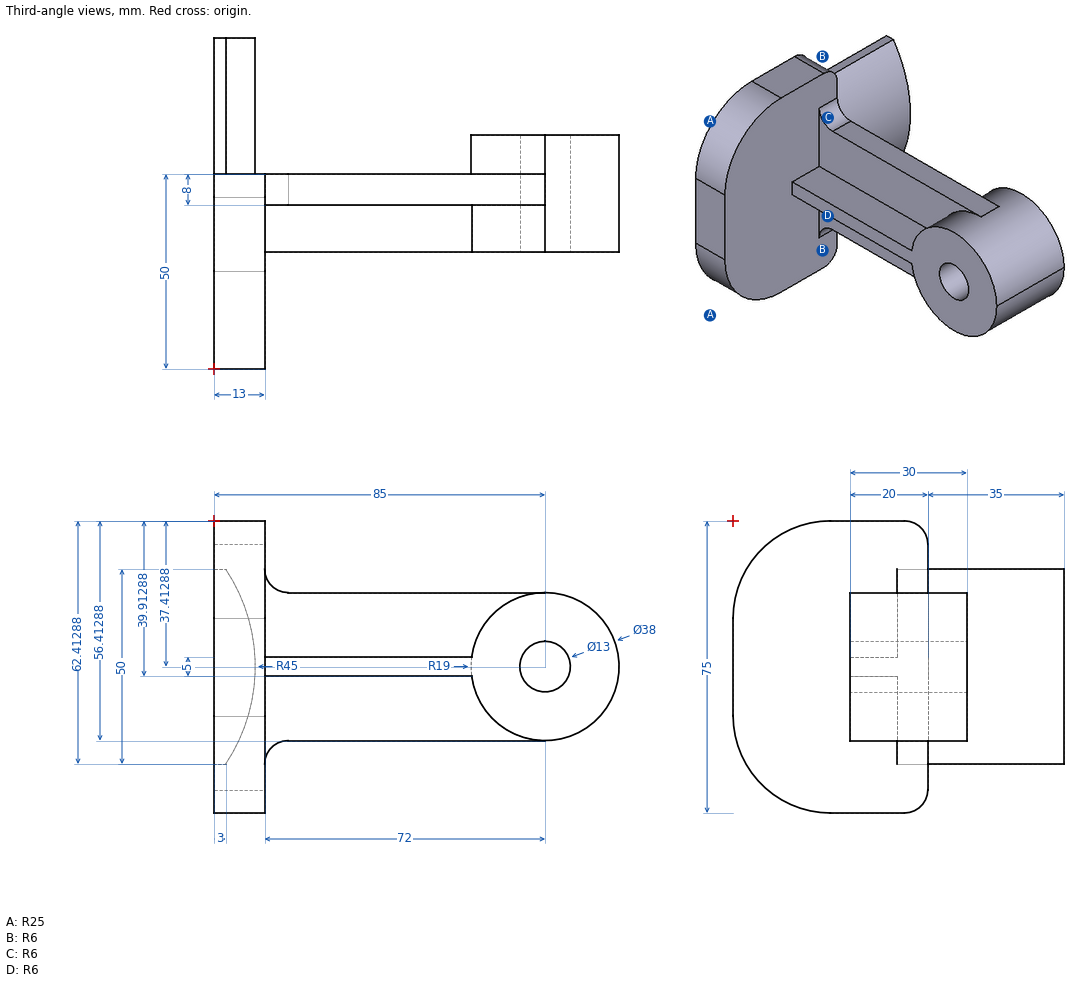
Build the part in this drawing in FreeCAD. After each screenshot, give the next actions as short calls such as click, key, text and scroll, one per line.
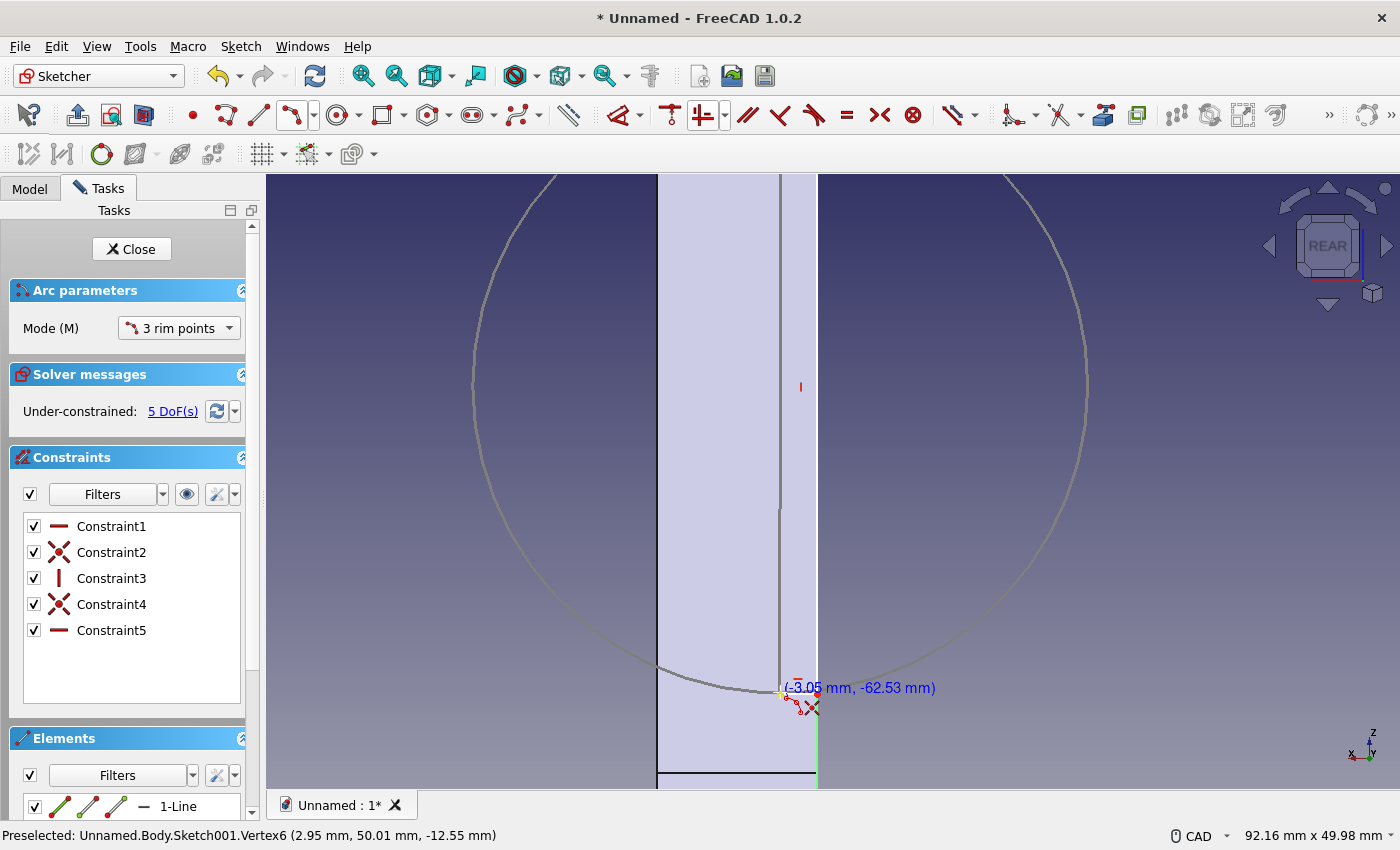
click(781, 694)
click(687, 384)
key(Escape)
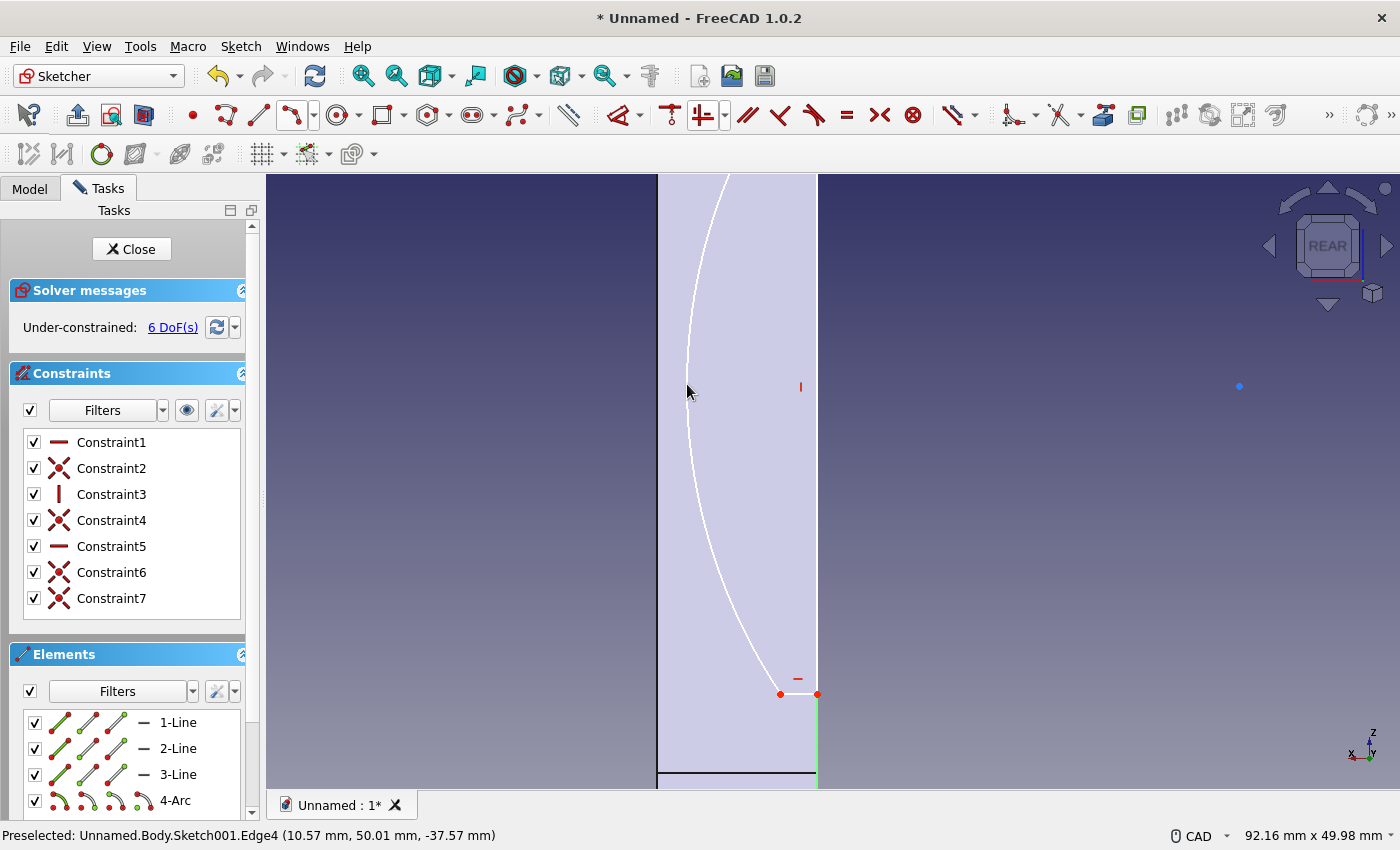
click(618, 116)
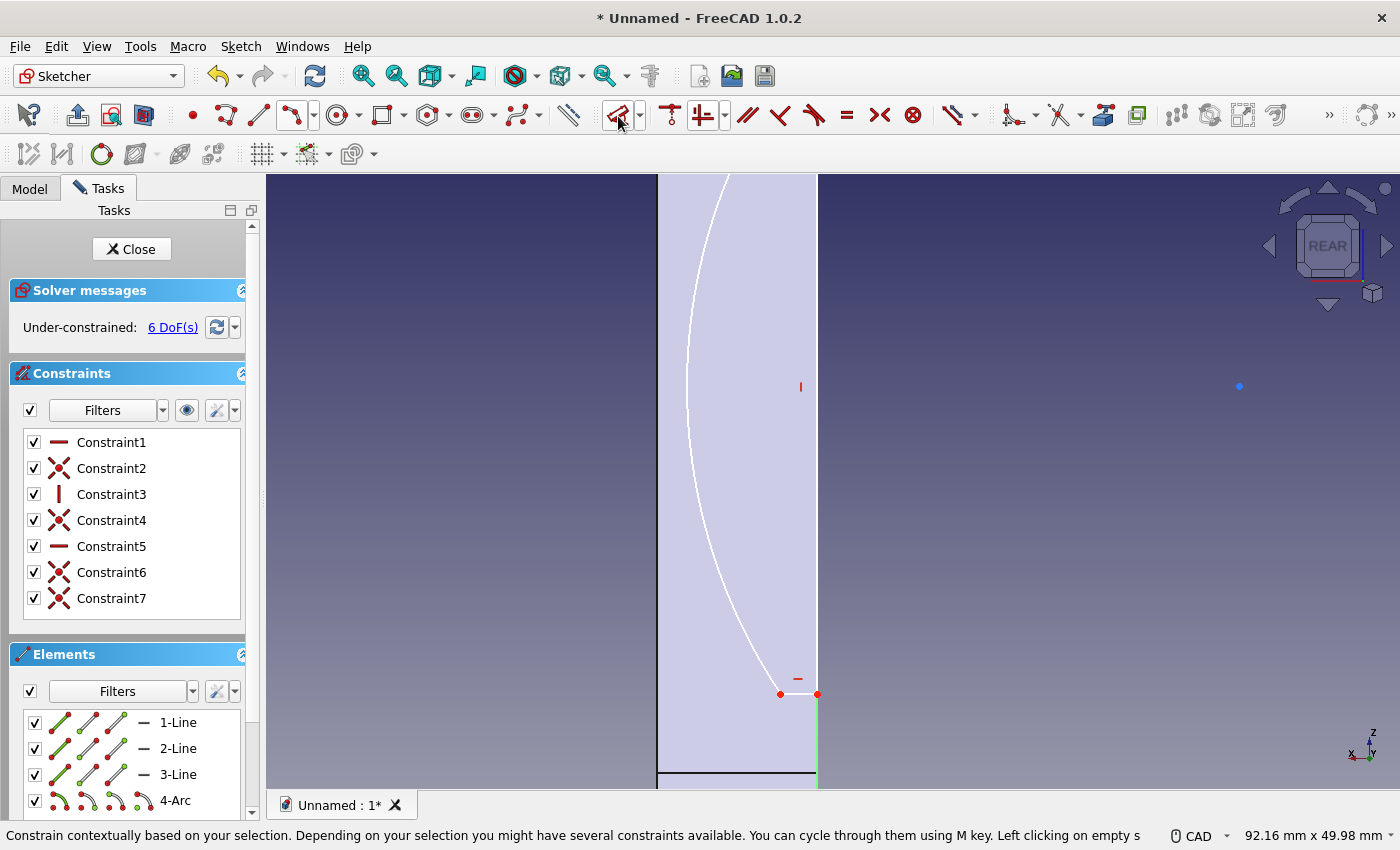
click(702, 257)
click(671, 250)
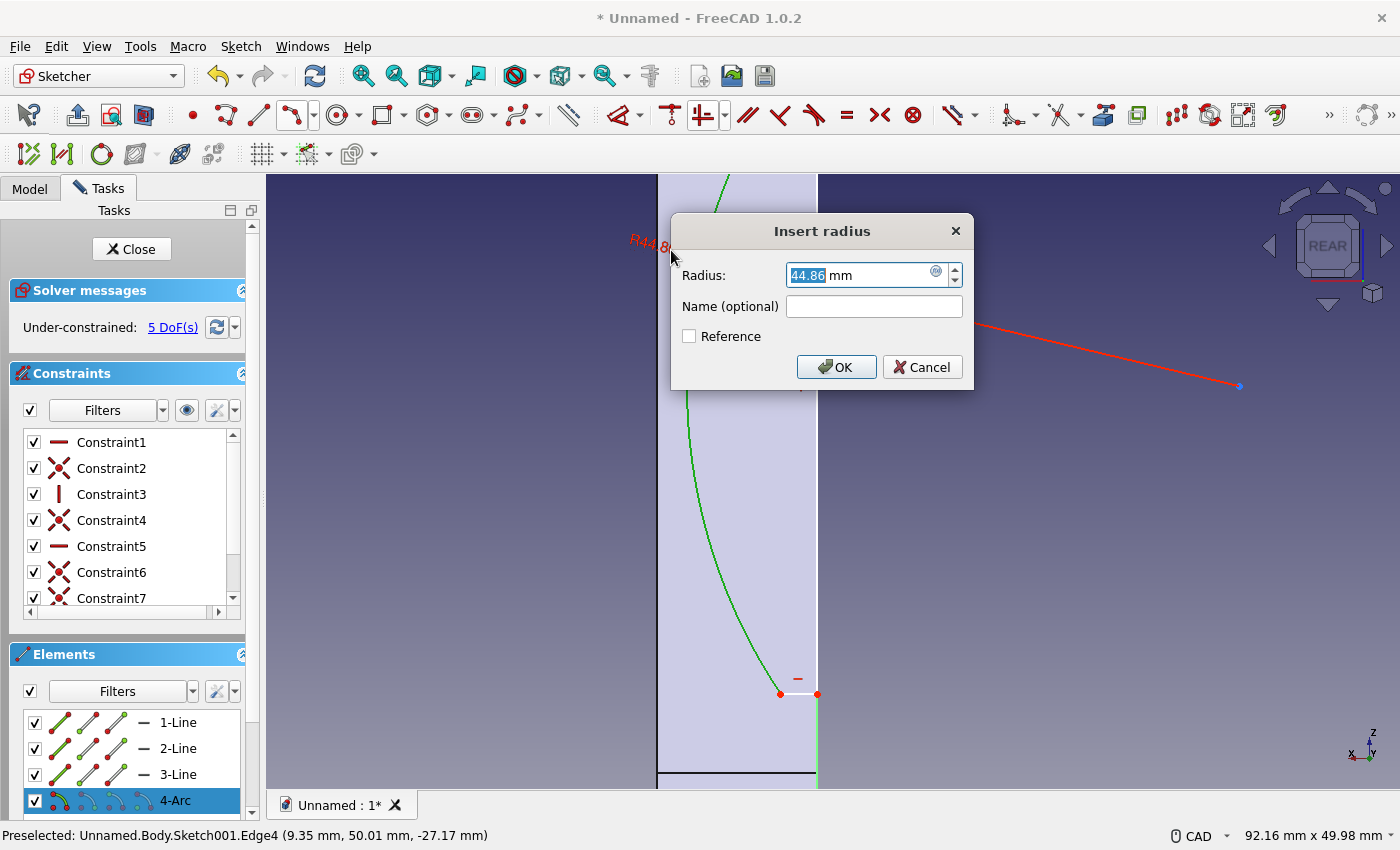
text(45)
key(Return)
key(Escape)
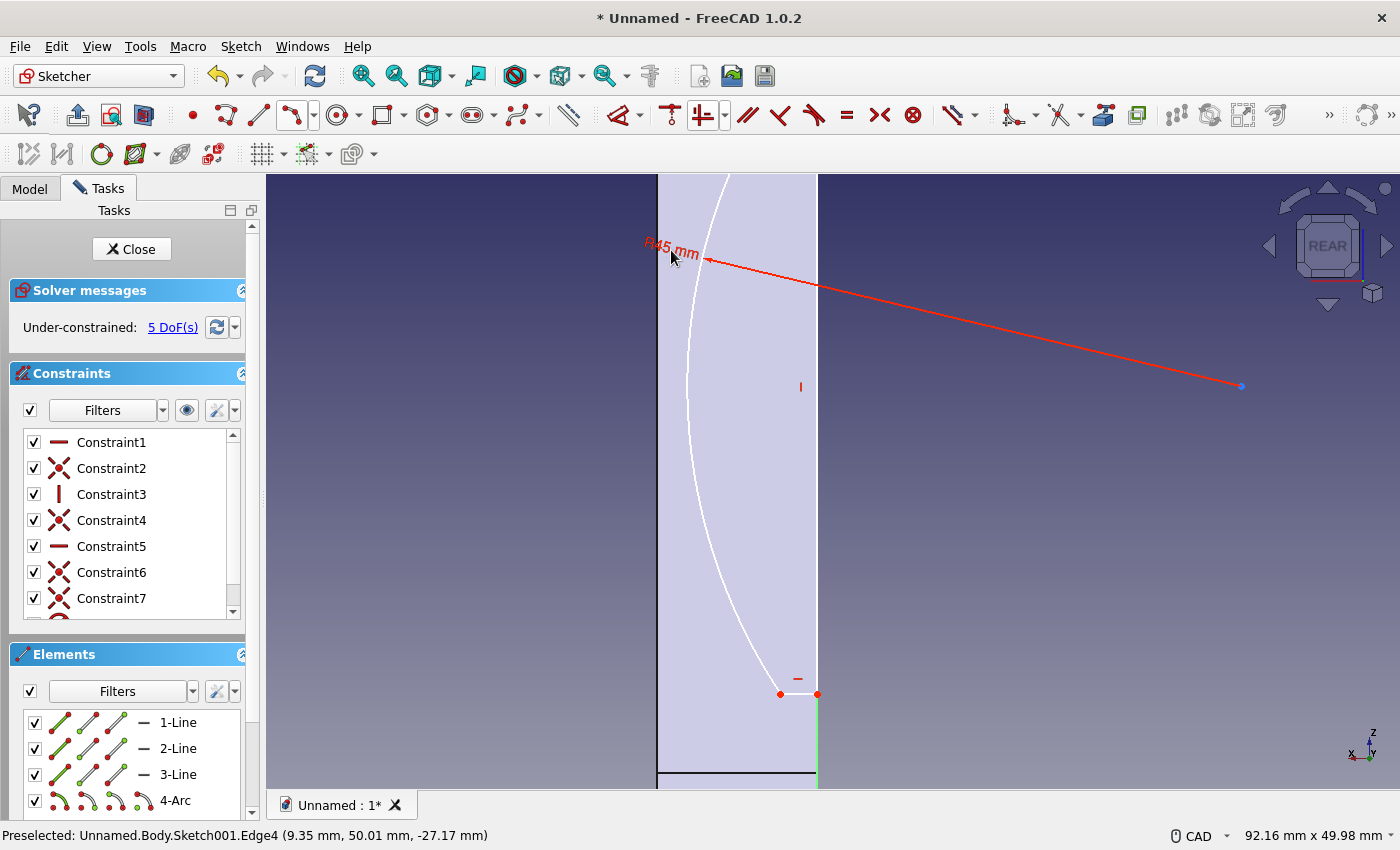
click(817, 694)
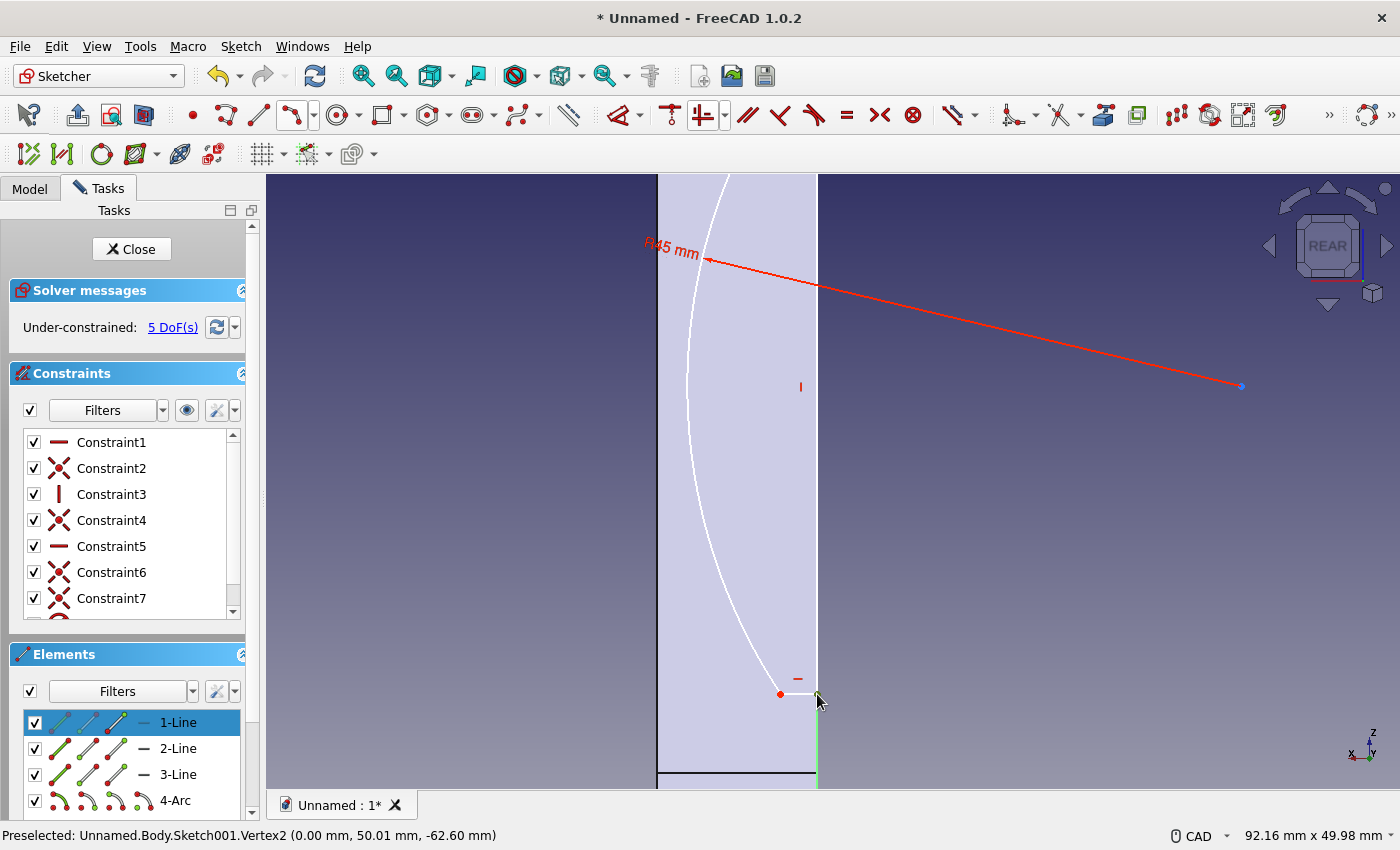
click(817, 721)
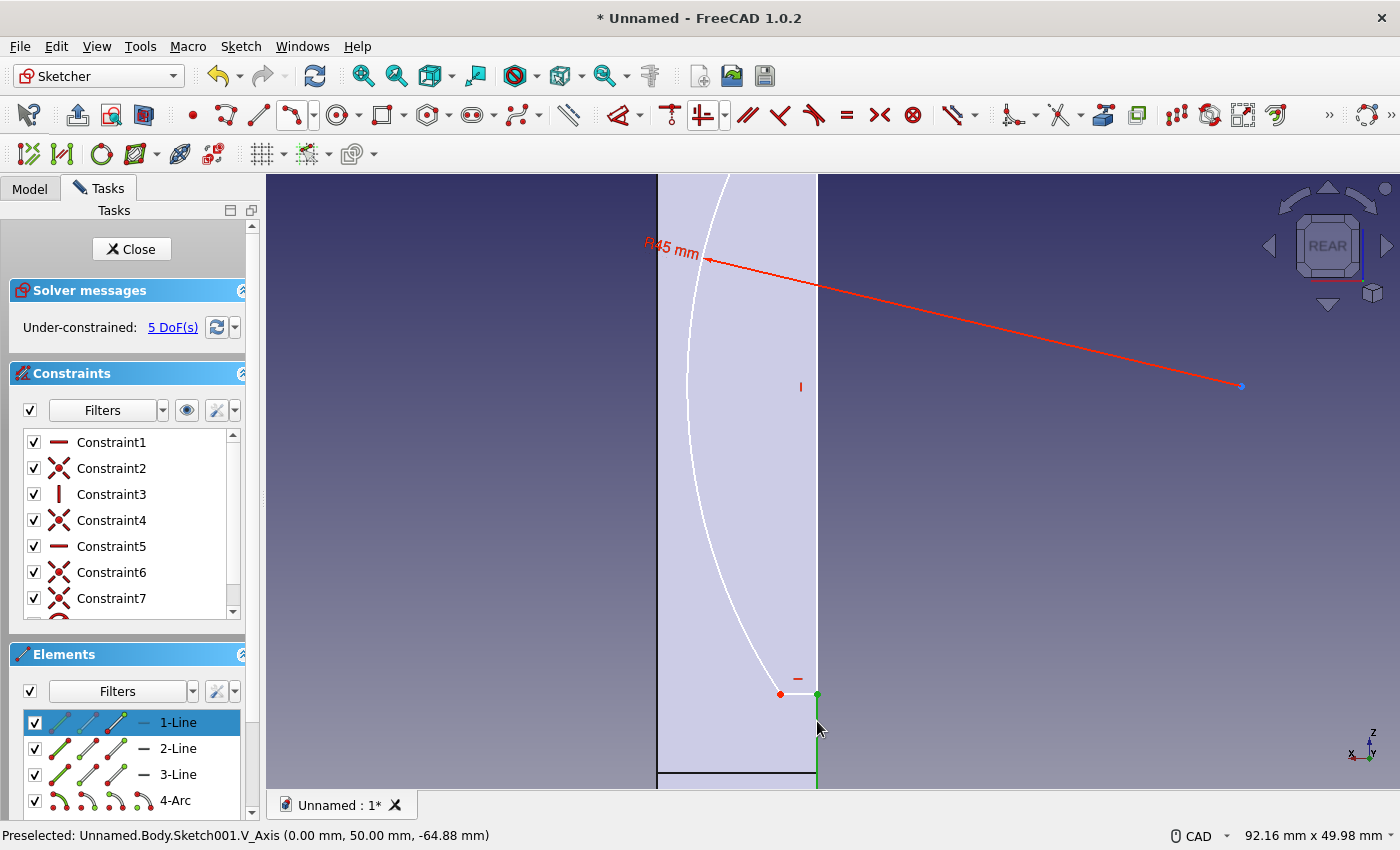
click(670, 116)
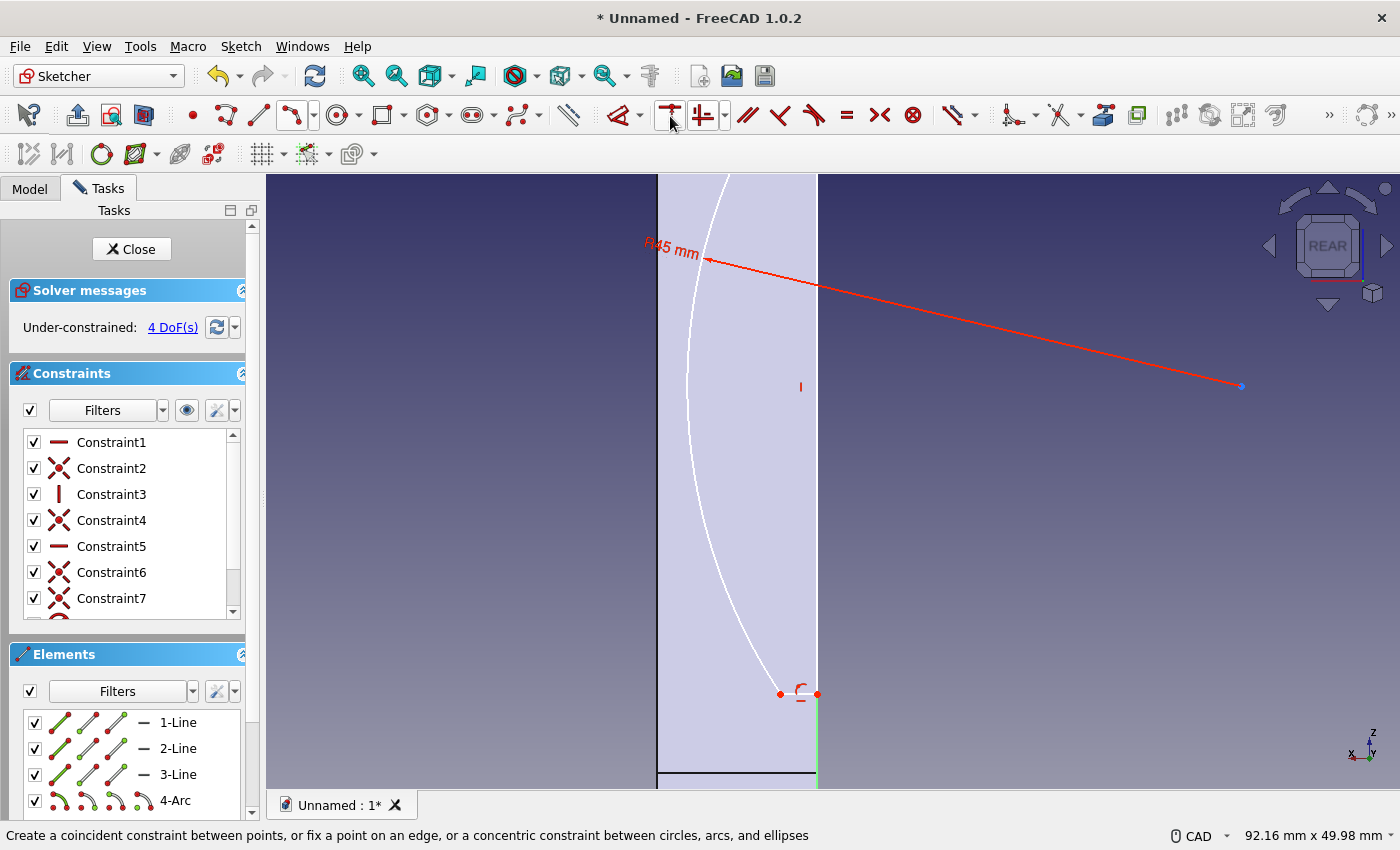
click(618, 116)